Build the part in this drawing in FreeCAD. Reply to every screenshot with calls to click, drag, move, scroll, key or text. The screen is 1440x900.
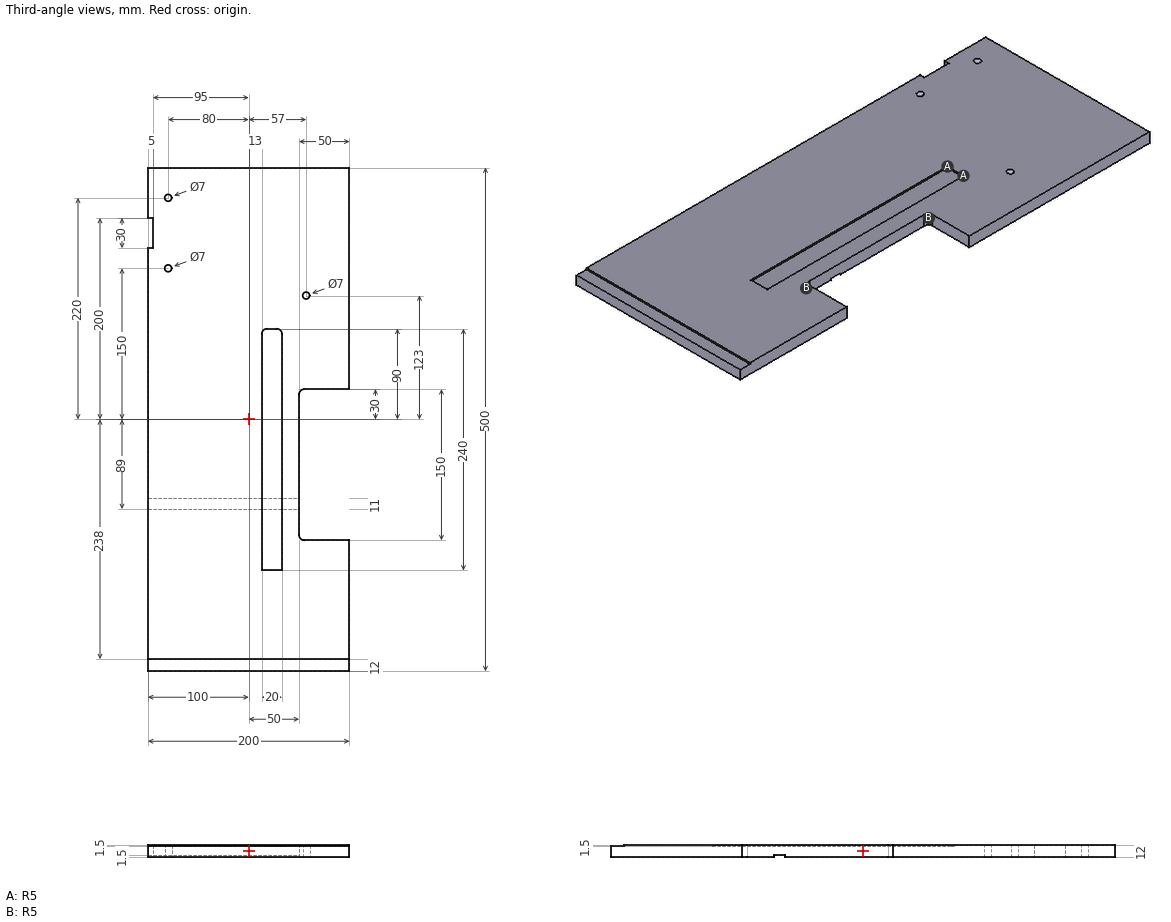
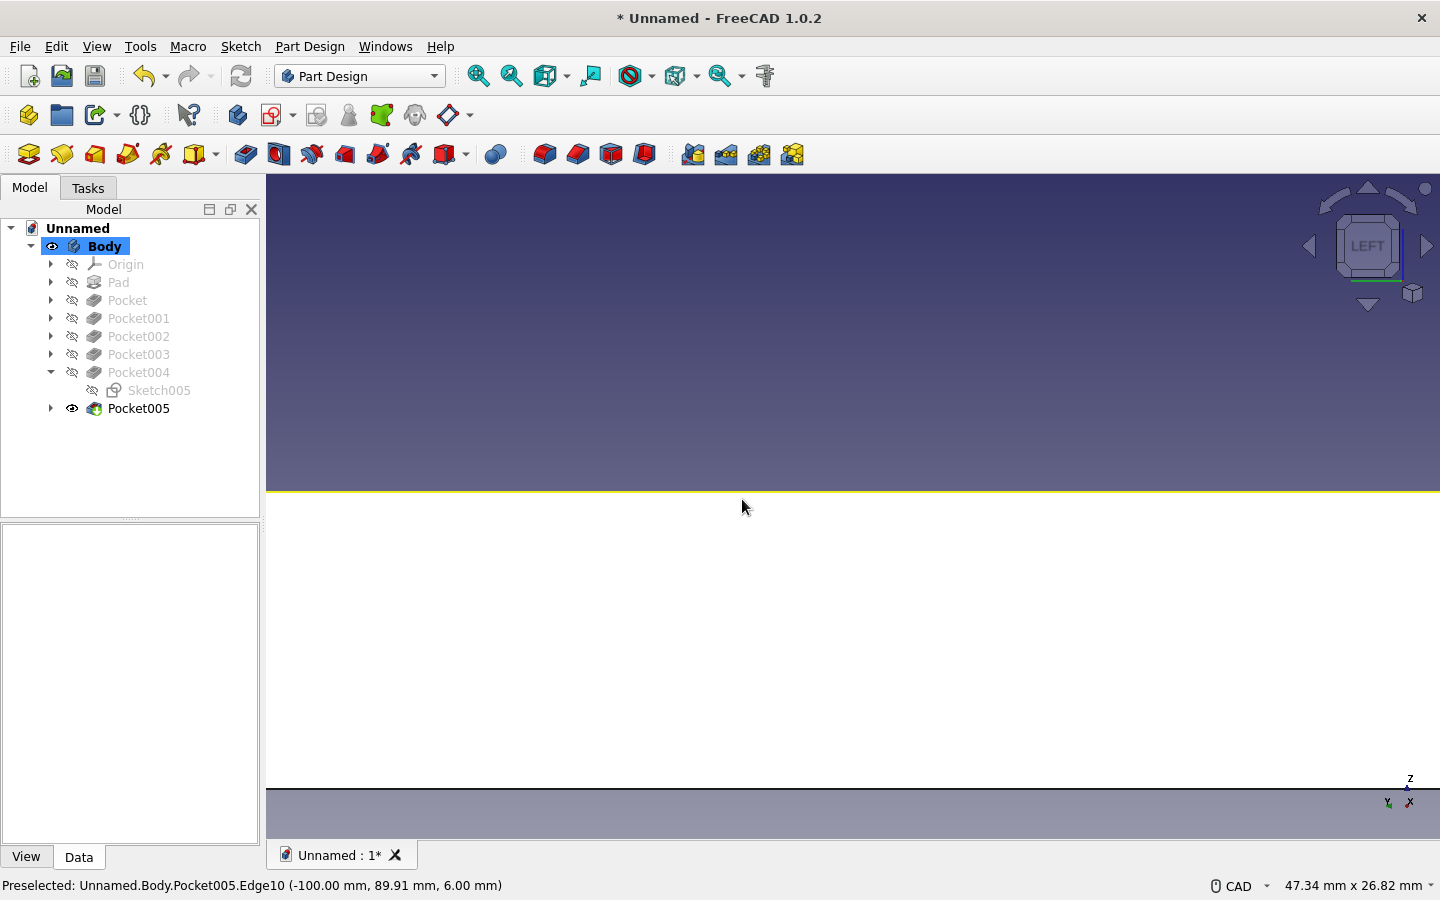
click(479, 76)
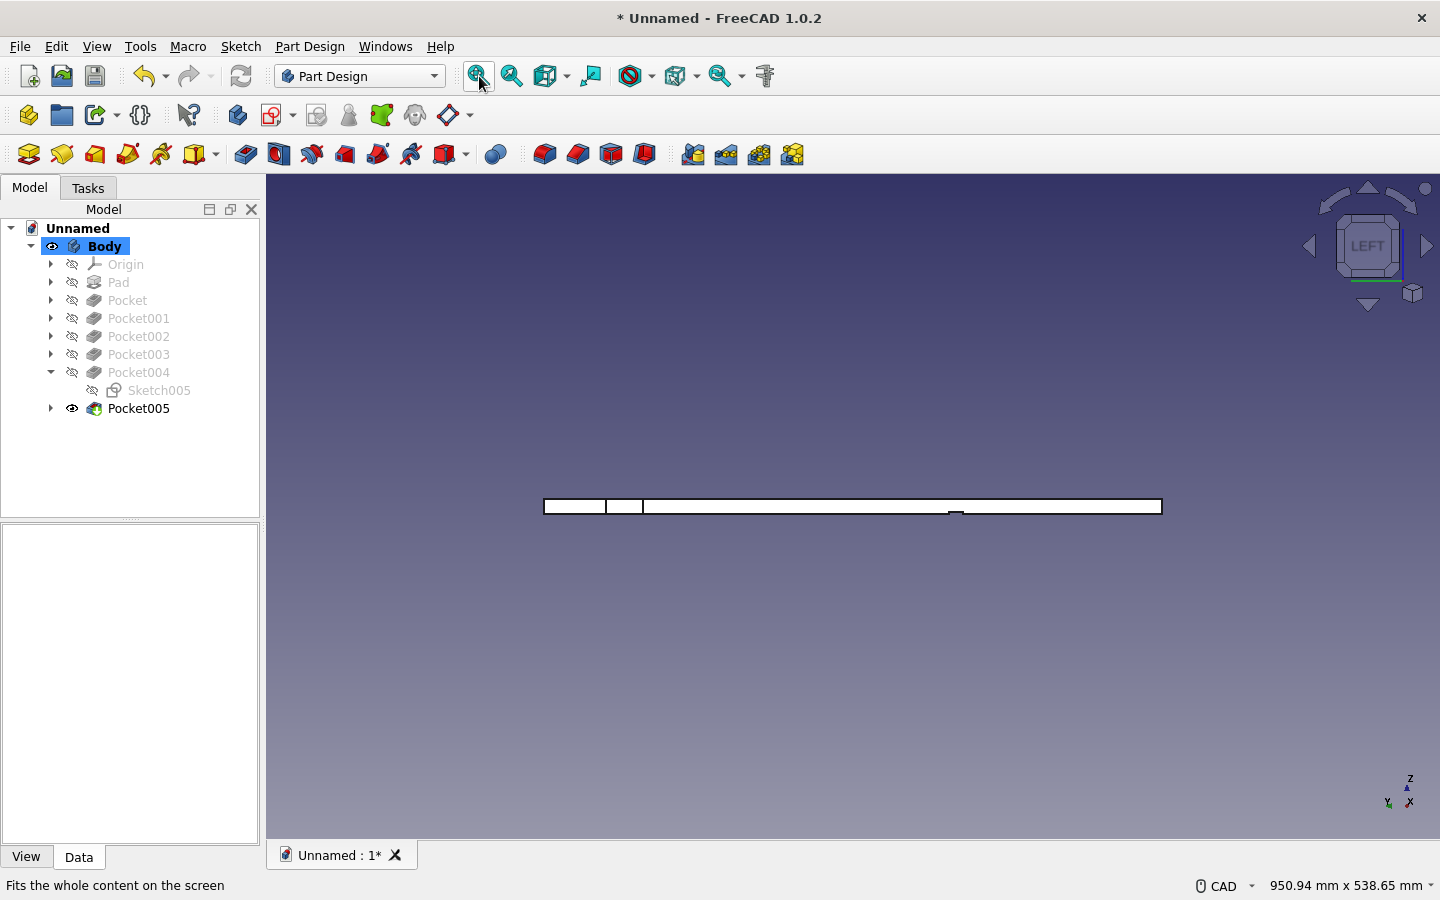
key(v)
key(3)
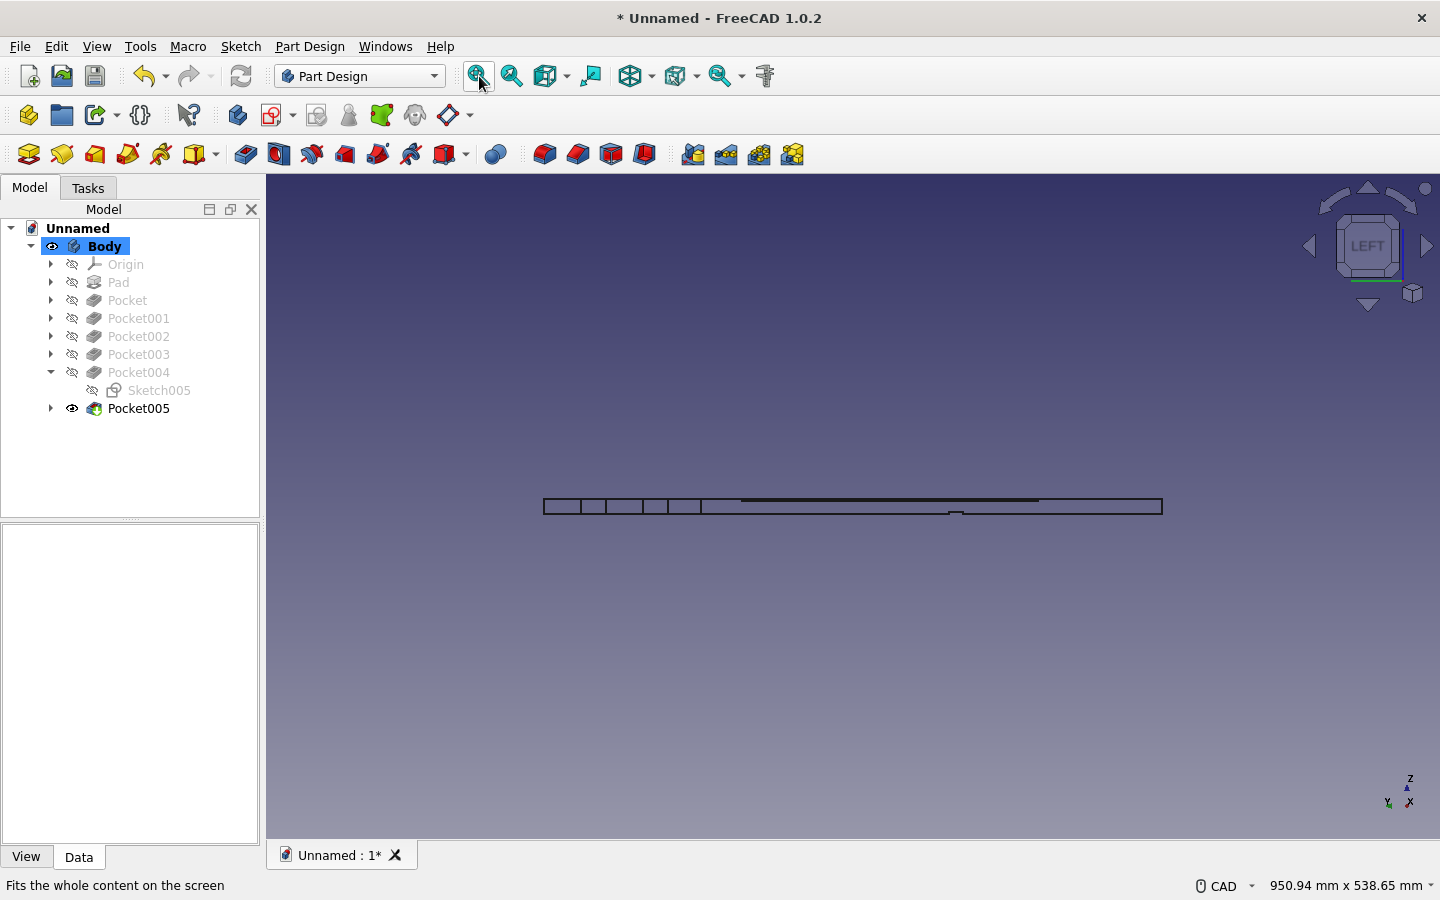
key(0)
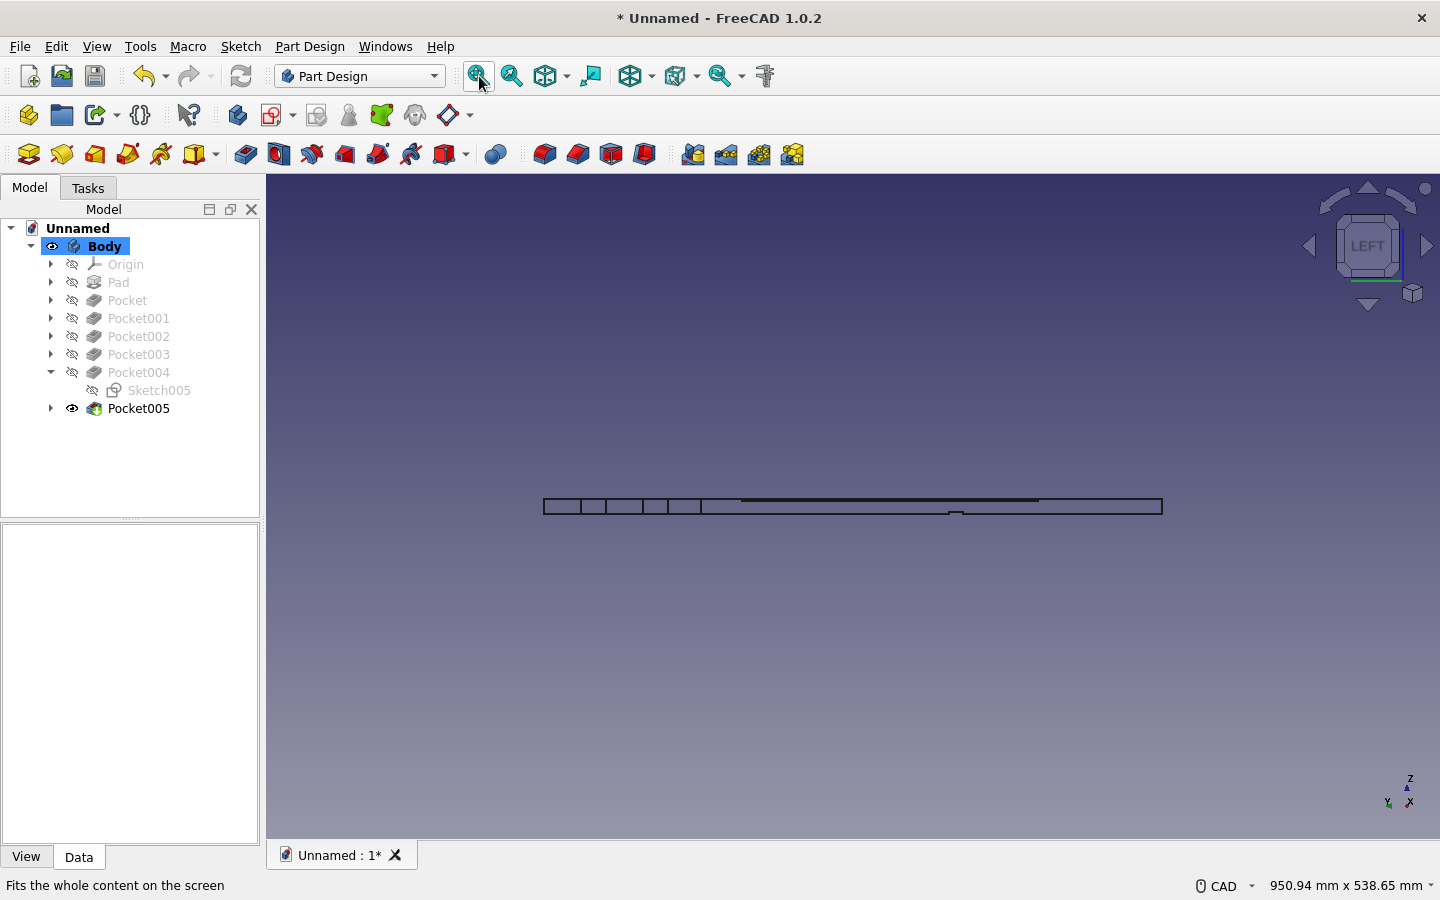
scroll(960, 471, up, 15)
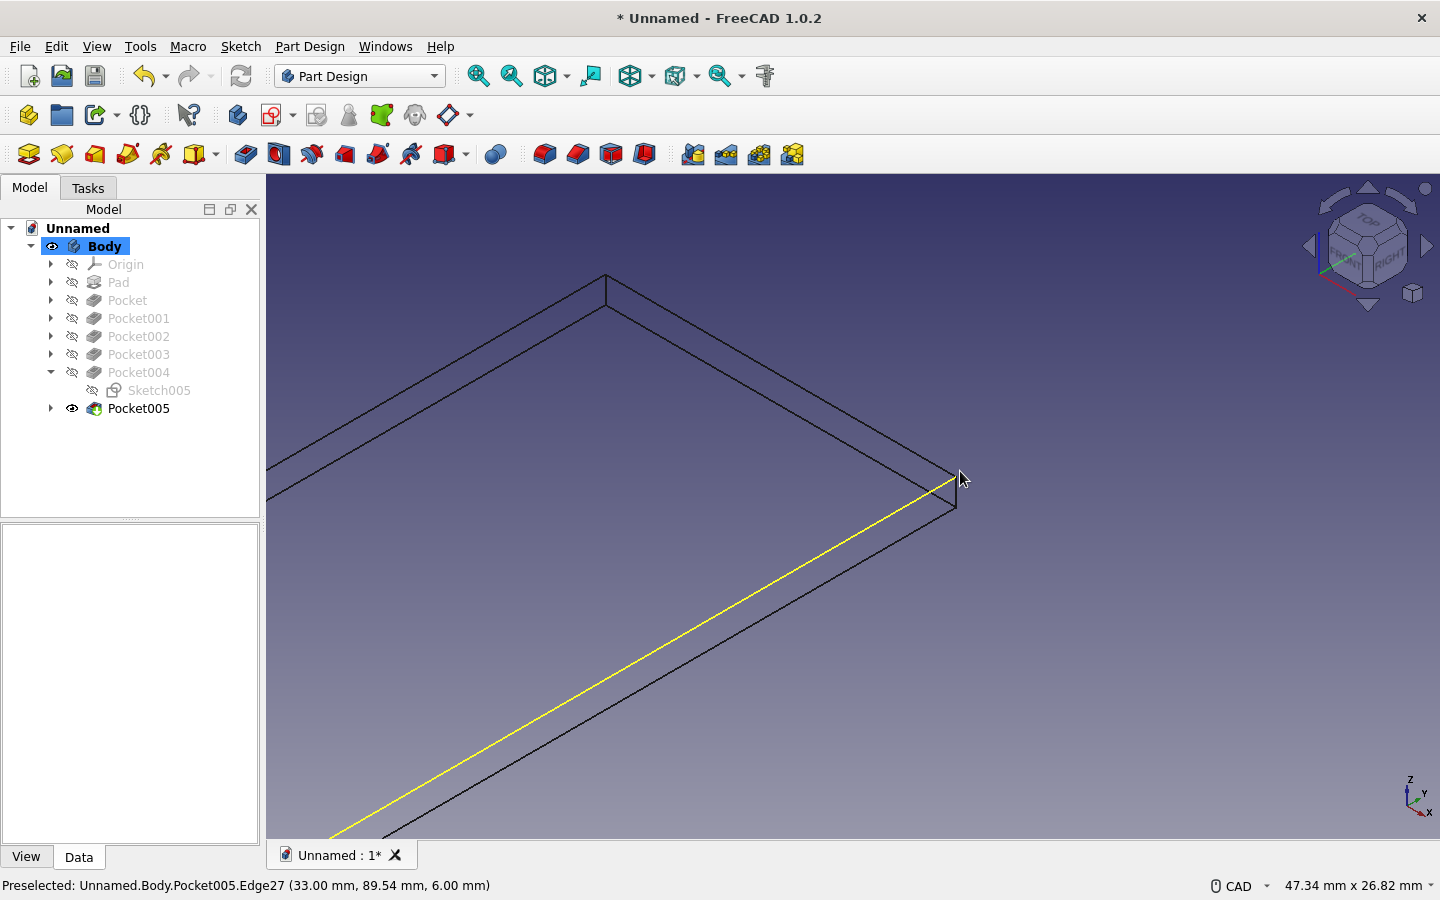
click(956, 491)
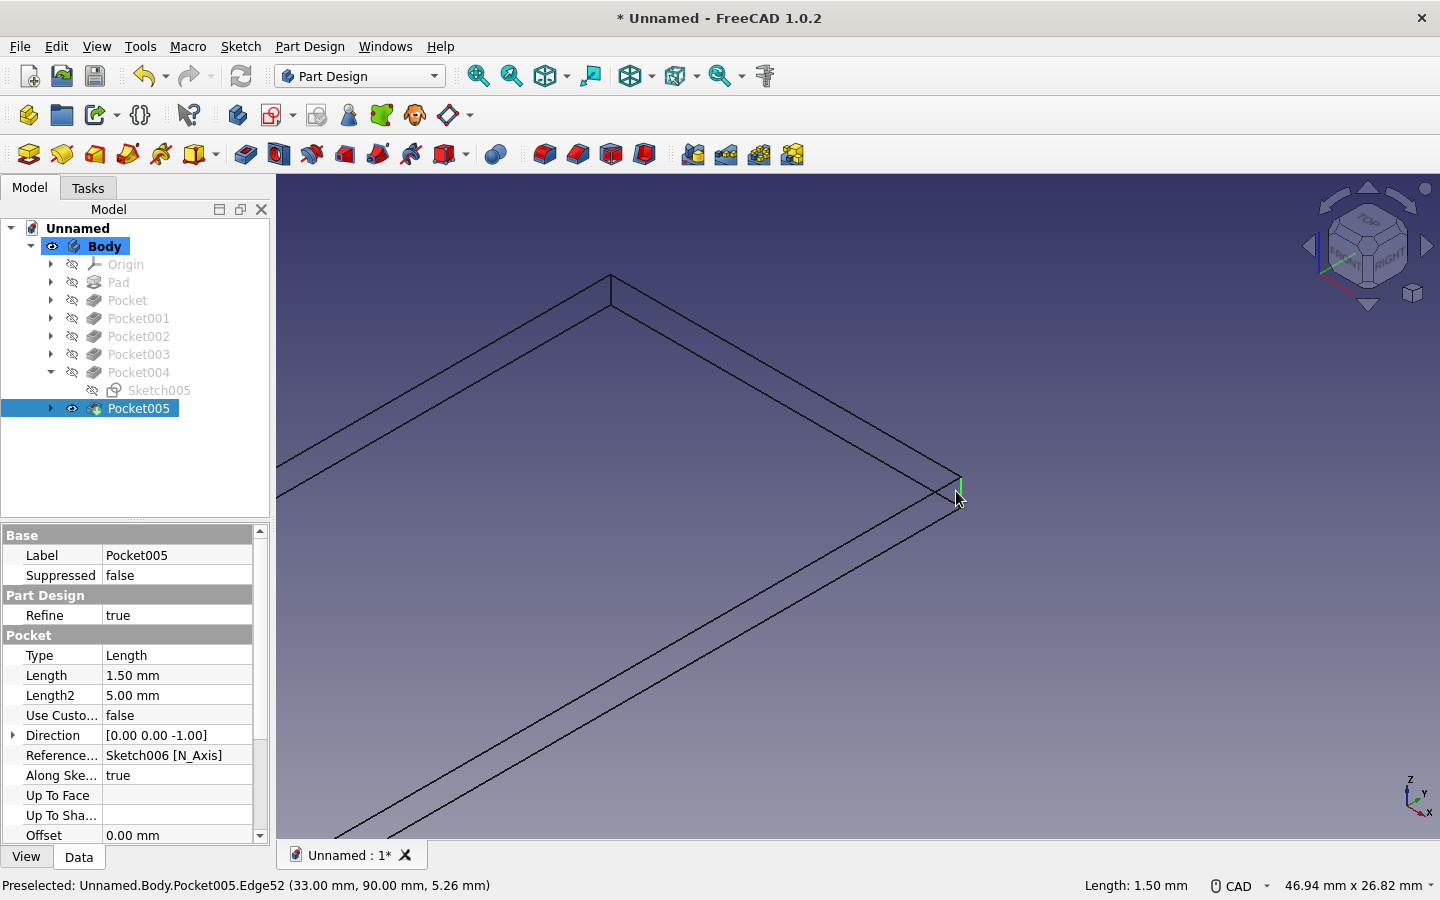
click(611, 289, ctrl)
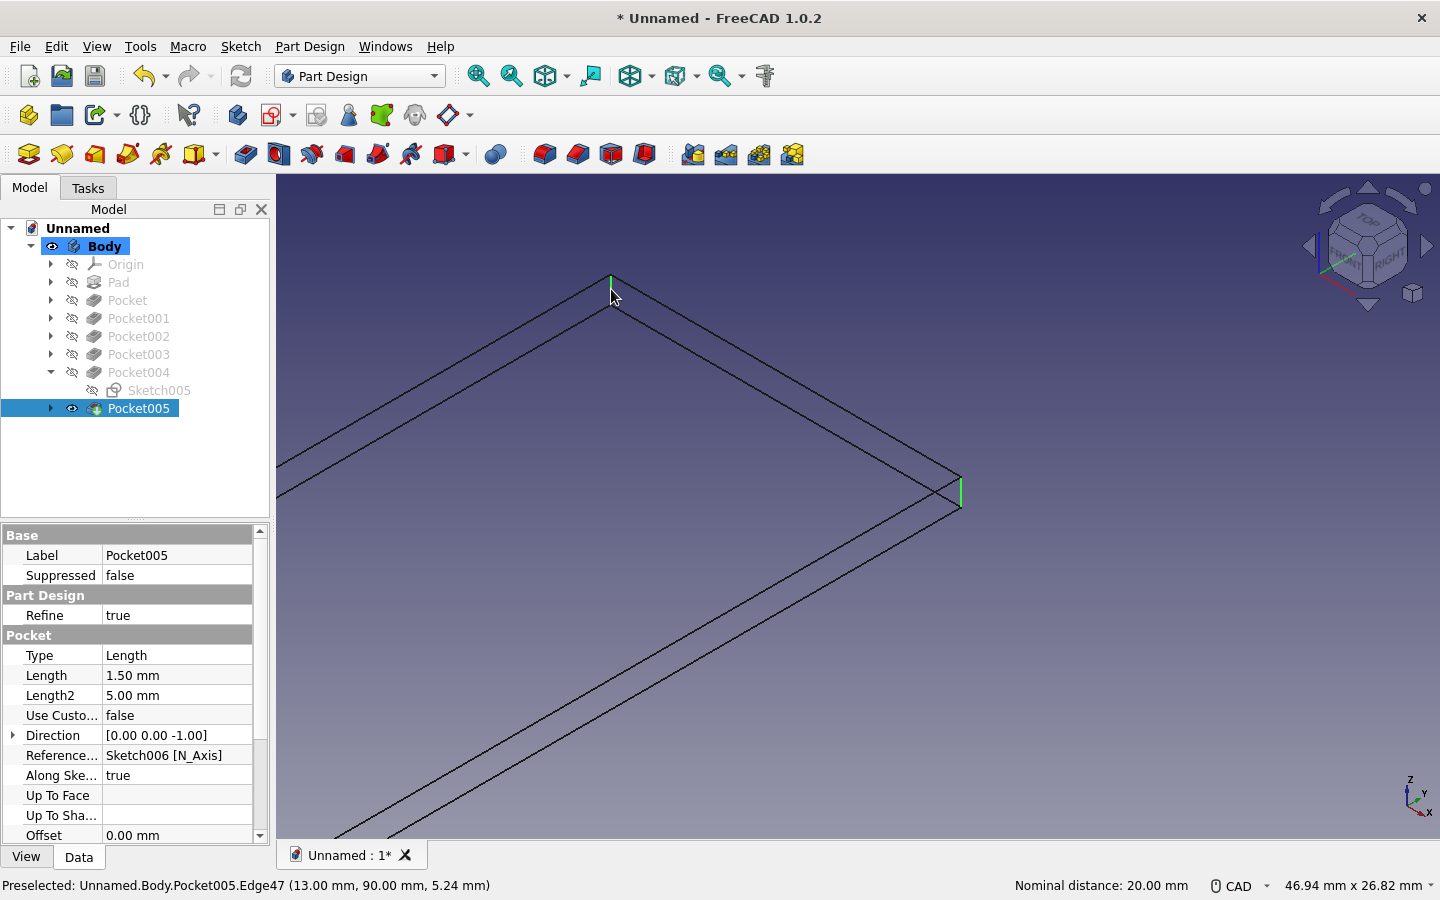
key(v)
key(1)